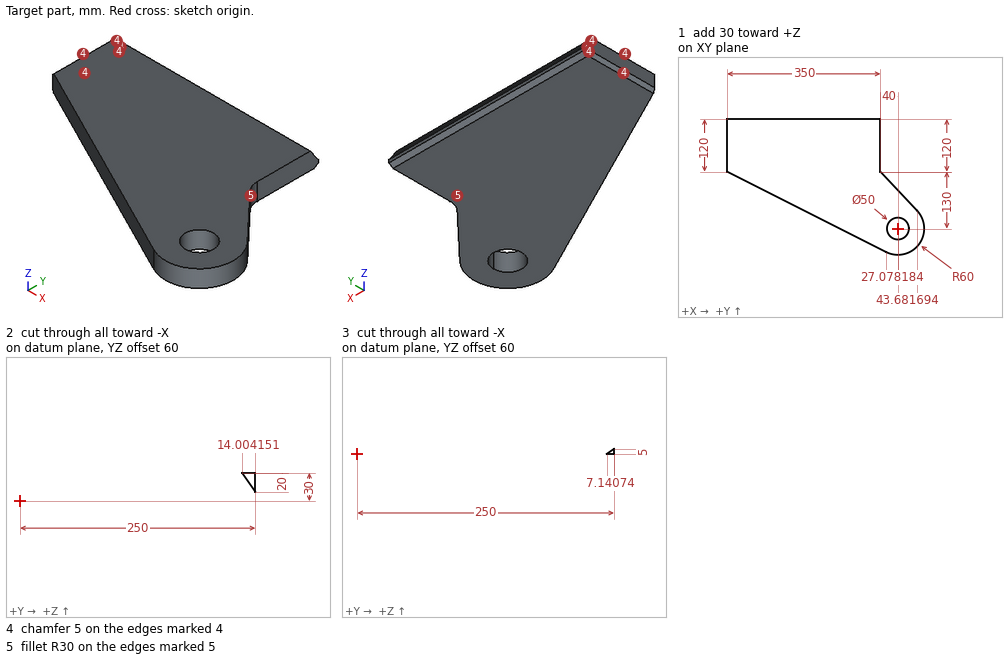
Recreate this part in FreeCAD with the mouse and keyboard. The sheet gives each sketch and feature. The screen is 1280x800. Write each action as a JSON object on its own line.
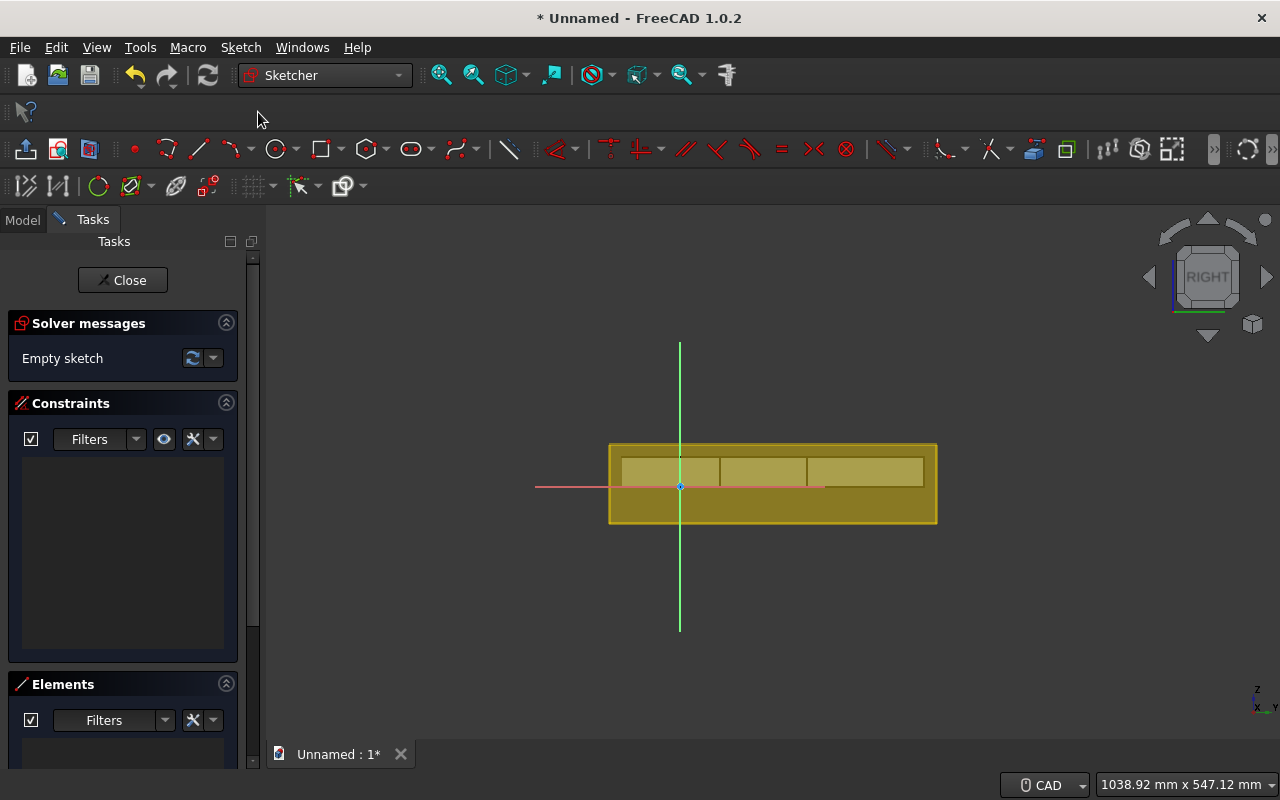
{"action": "scroll", "coordinate": [931, 467], "scroll_direction": "up", "scroll_amount": 14}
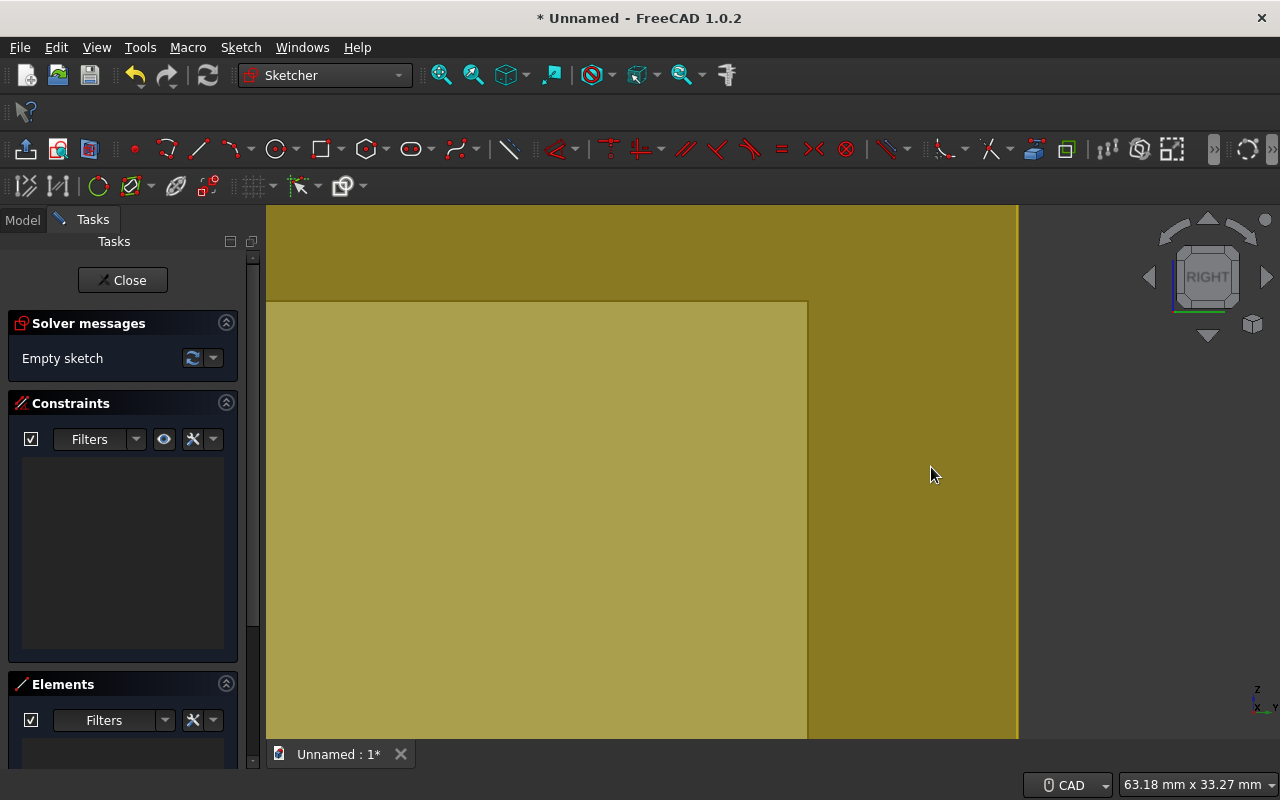
{"action": "left_click", "coordinate": [168, 150]}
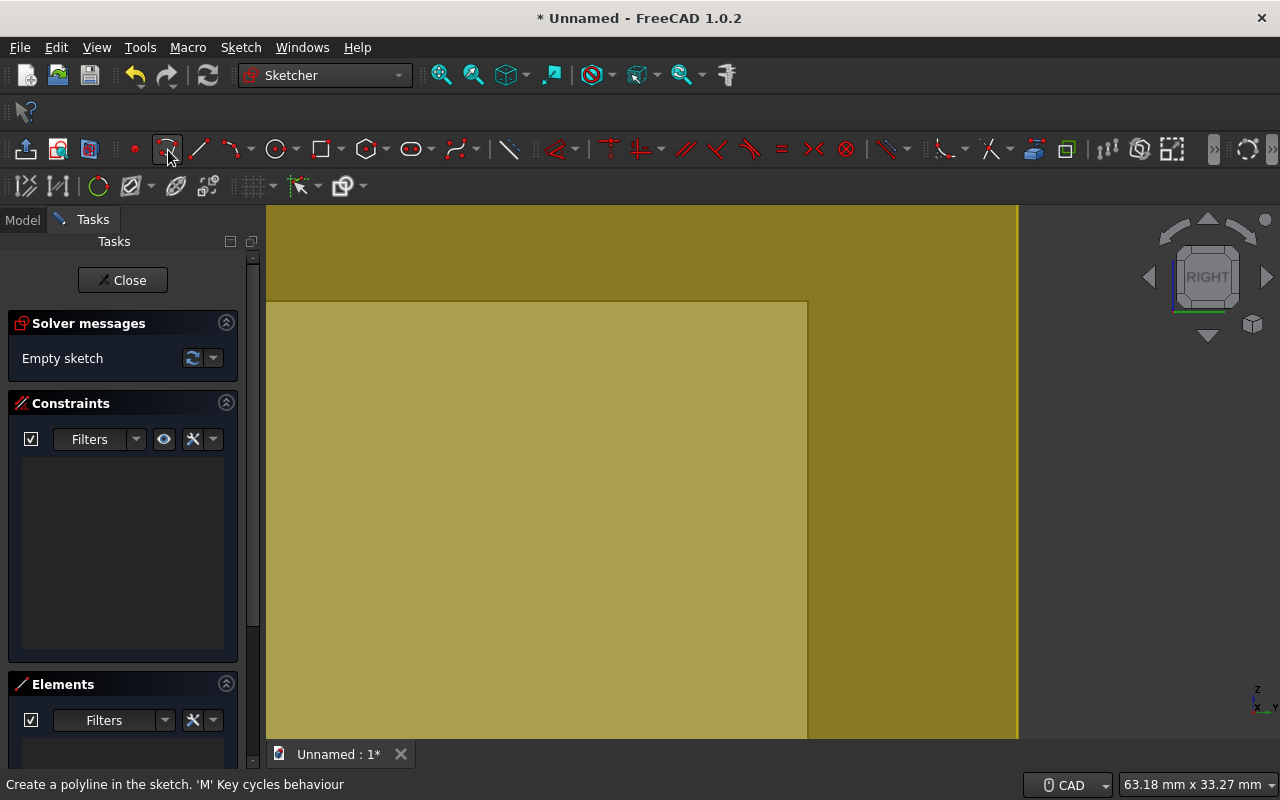
{"action": "left_click", "coordinate": [584, 301]}
{"action": "left_click", "coordinate": [808, 622]}
{"action": "left_click", "coordinate": [808, 301]}
{"action": "left_click", "coordinate": [584, 302]}
{"action": "key", "text": "Escape"}
{"action": "key", "text": "Escape"}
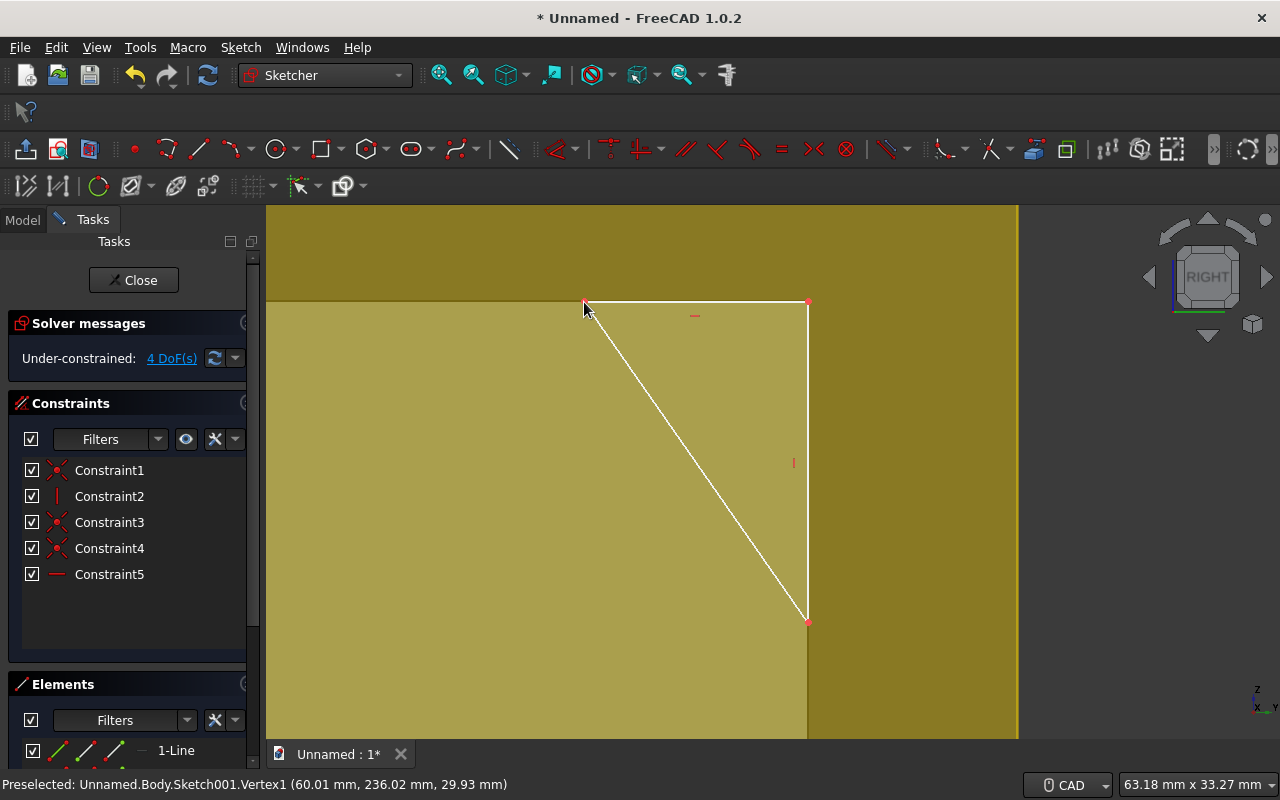
{"action": "left_click", "coordinate": [556, 150]}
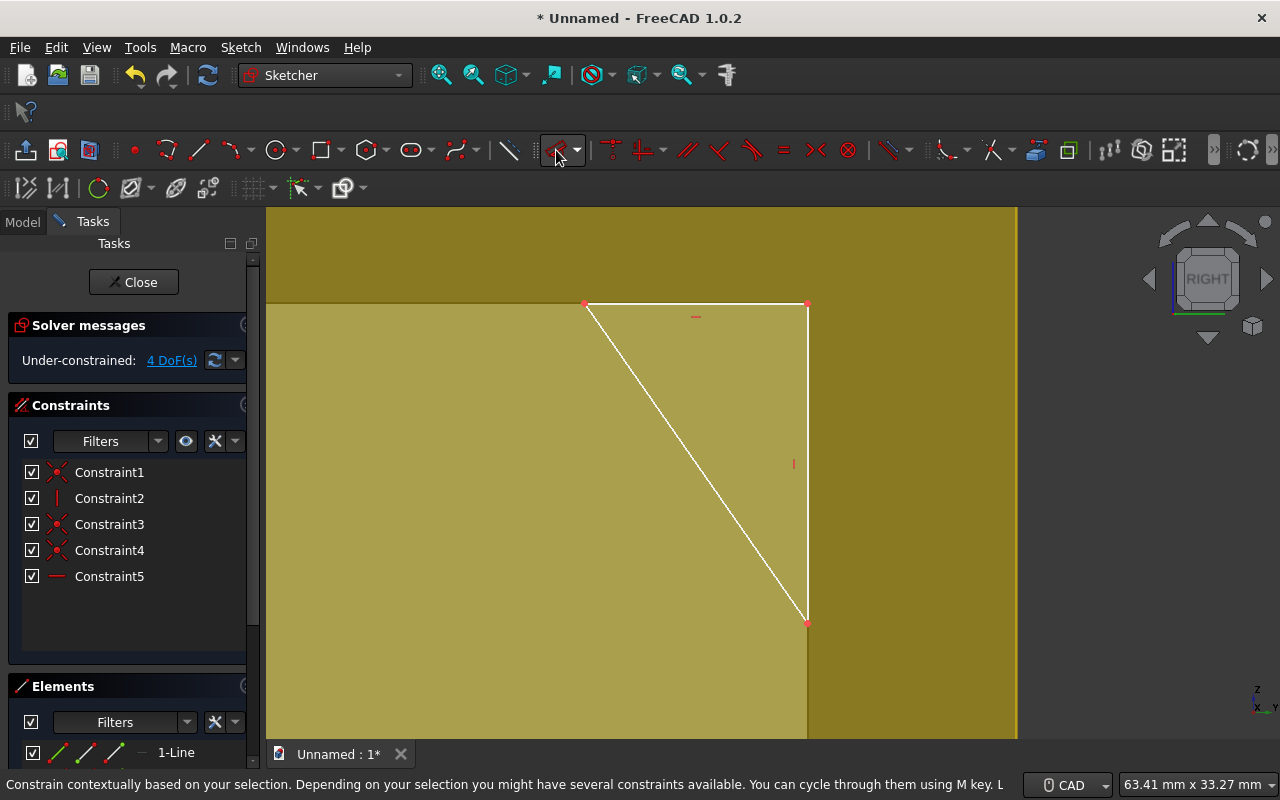
{"action": "left_click", "coordinate": [808, 527]}
{"action": "left_click", "coordinate": [842, 464]}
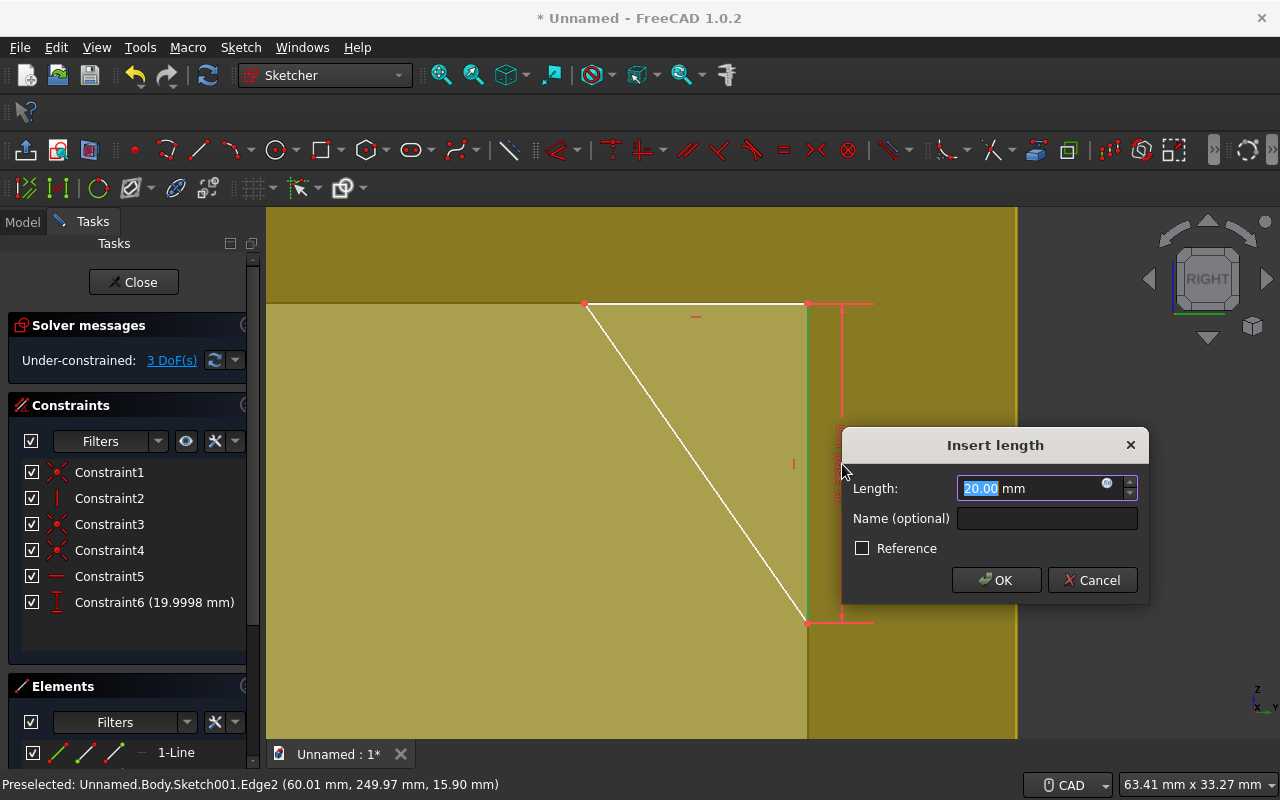
{"action": "type", "text": "20"}
{"action": "key", "text": "Return"}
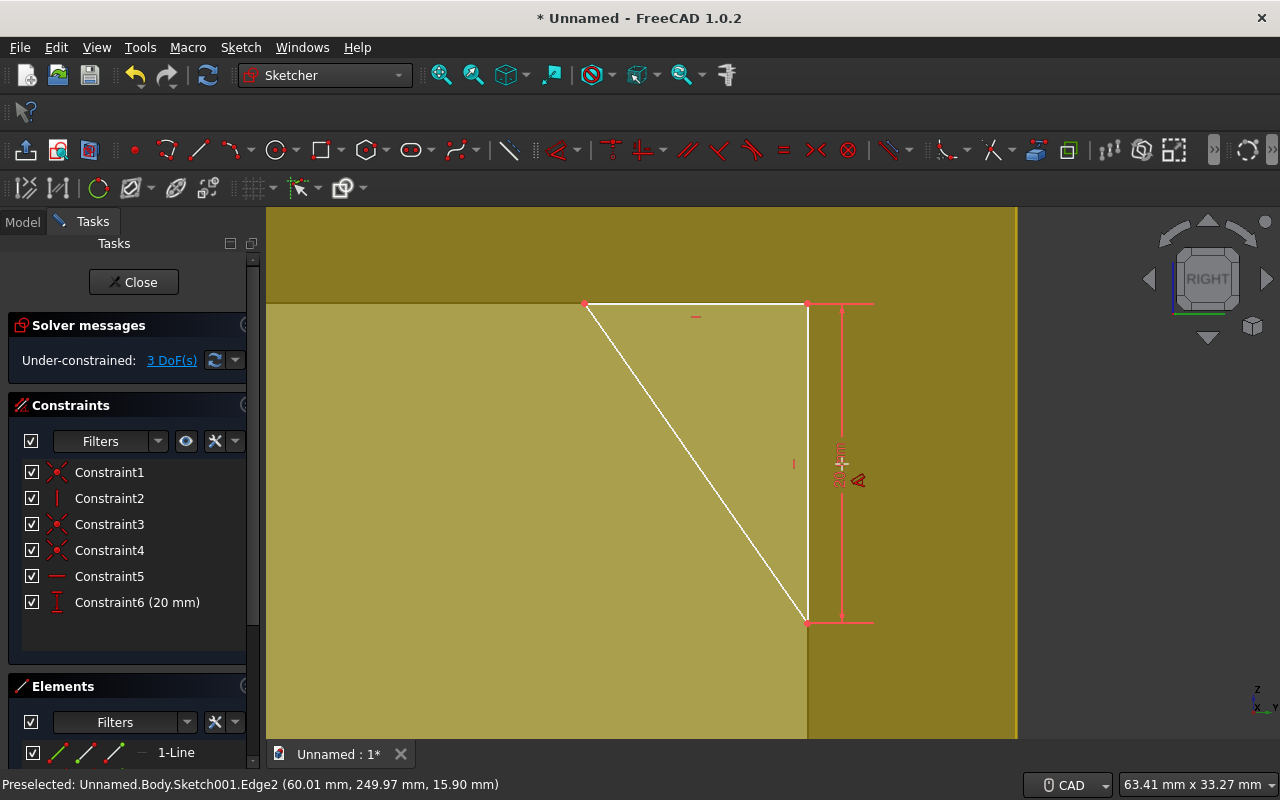
{"action": "left_click", "coordinate": [585, 304]}
{"action": "left_click", "coordinate": [619, 507]}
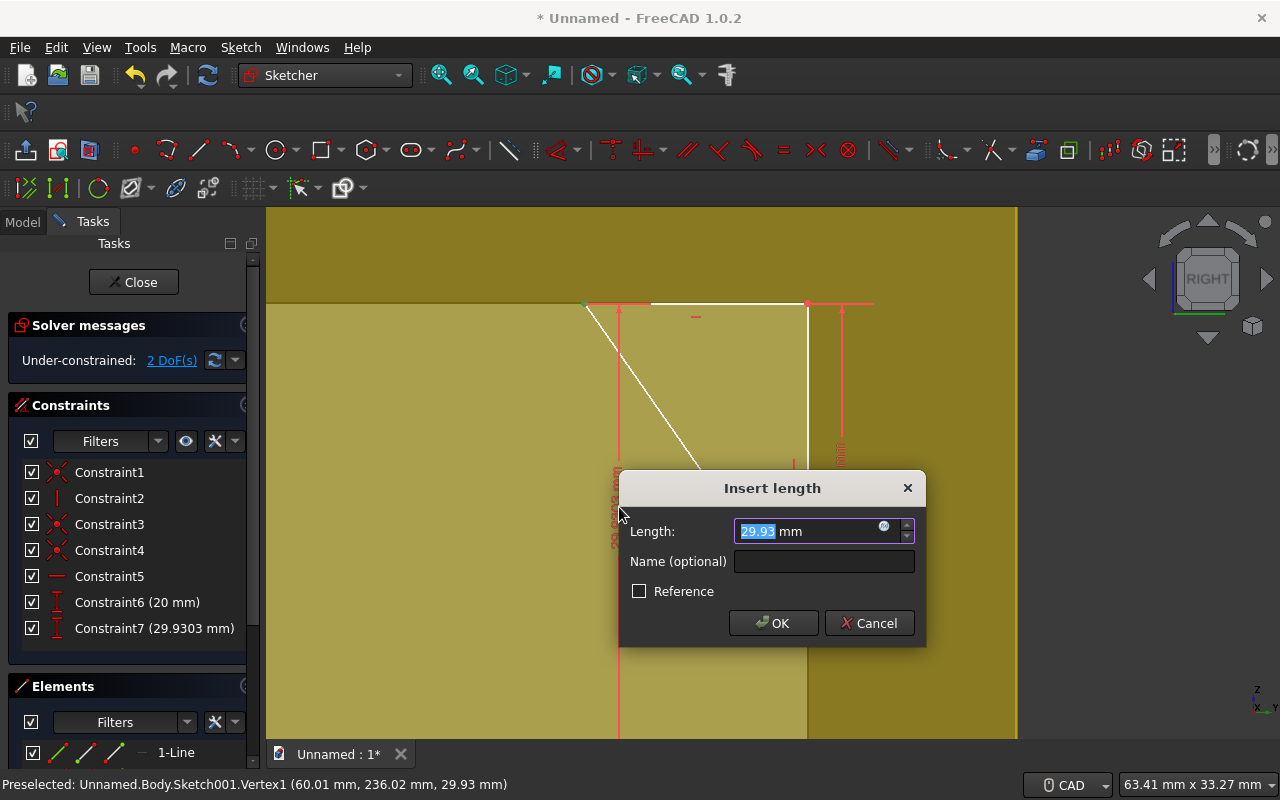
{"action": "type", "text": "30"}
{"action": "key", "text": "Return"}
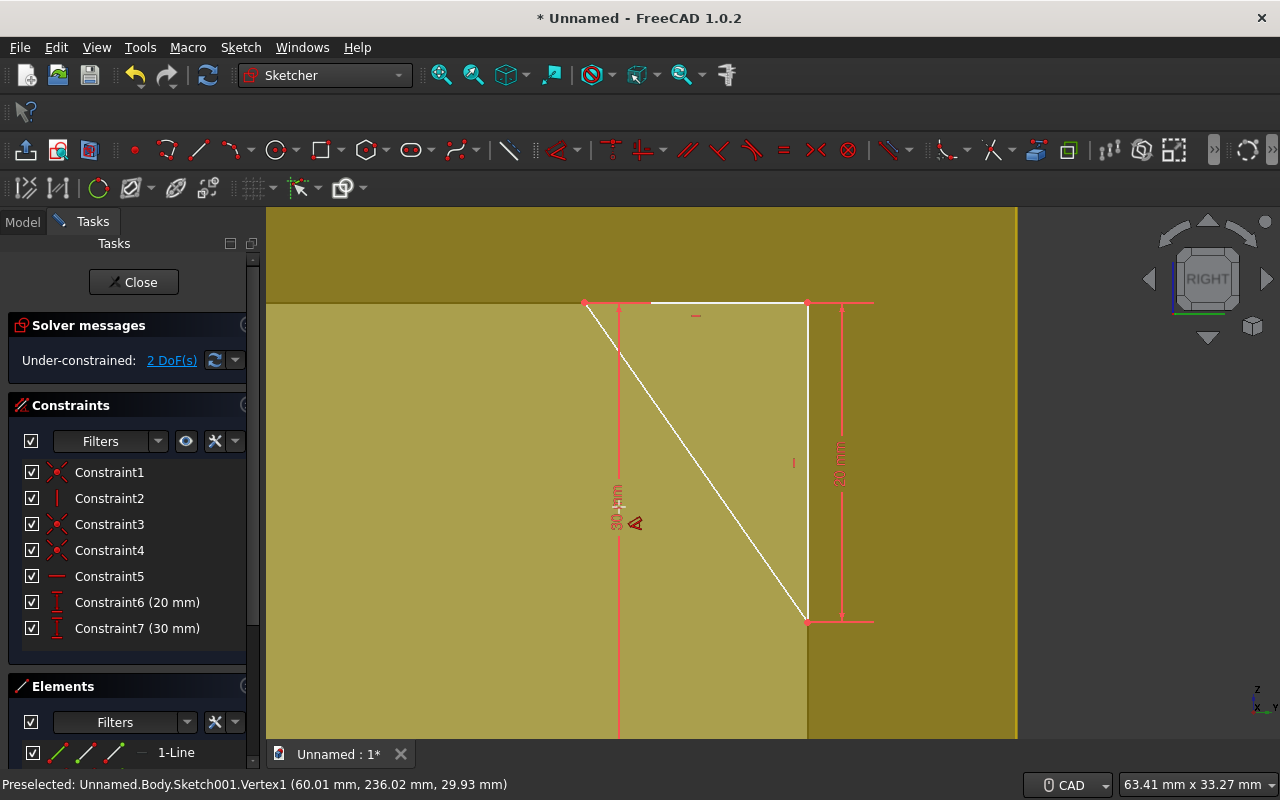
{"action": "left_click", "coordinate": [808, 622]}
{"action": "left_click", "coordinate": [551, 588]}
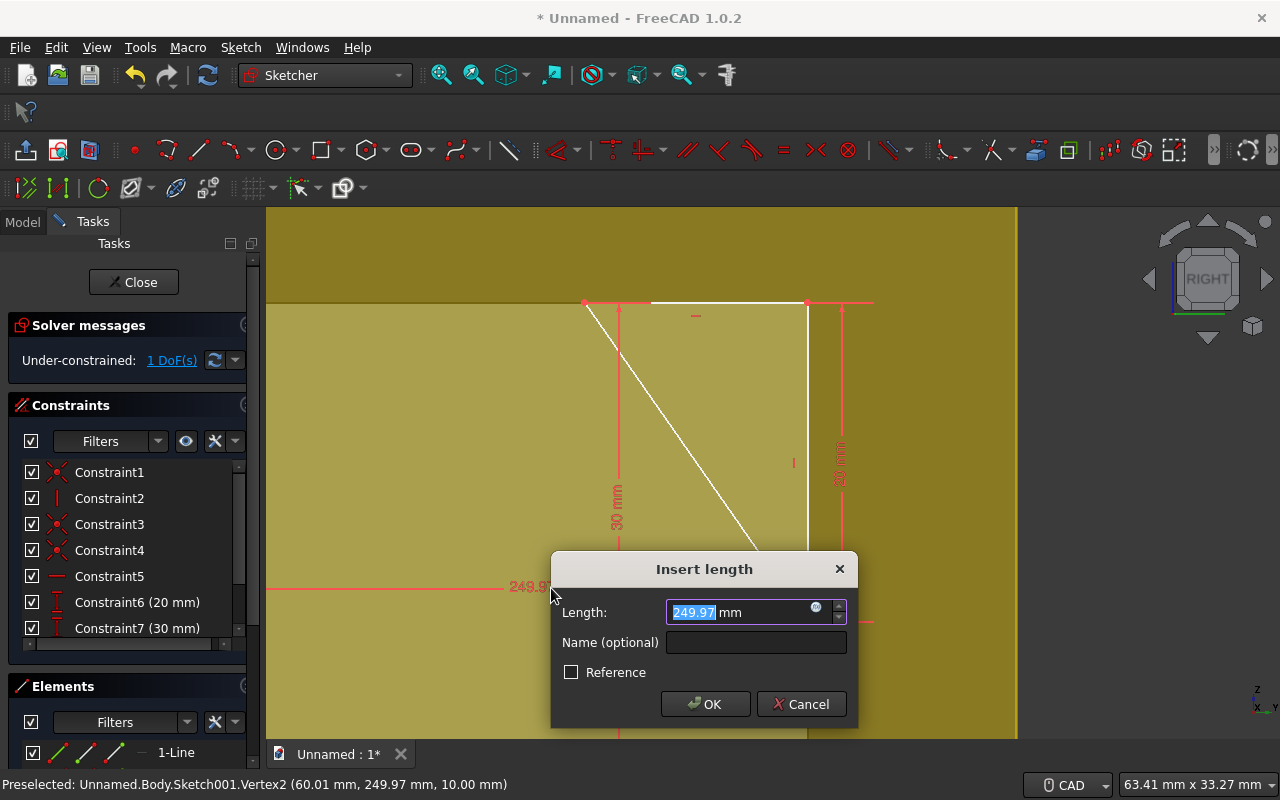
{"action": "type", "text": "250"}
{"action": "key", "text": "Return"}